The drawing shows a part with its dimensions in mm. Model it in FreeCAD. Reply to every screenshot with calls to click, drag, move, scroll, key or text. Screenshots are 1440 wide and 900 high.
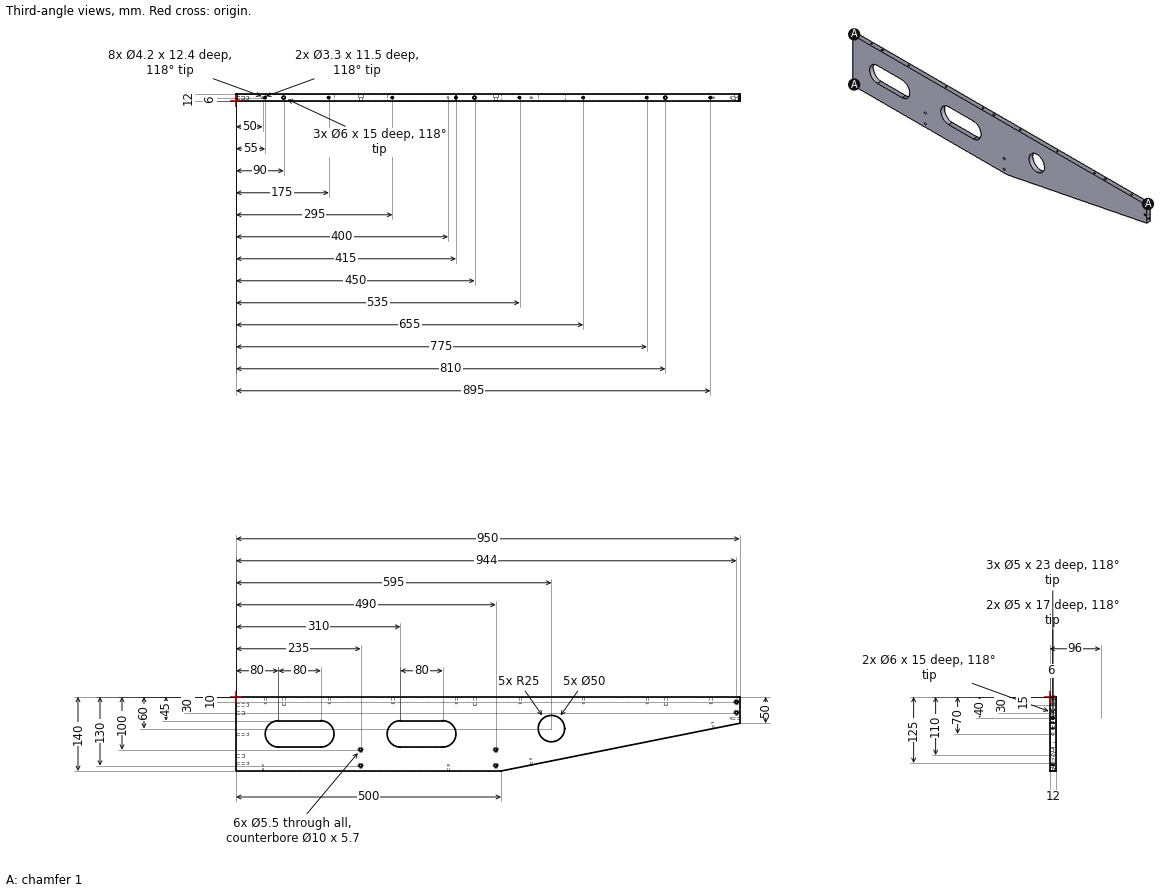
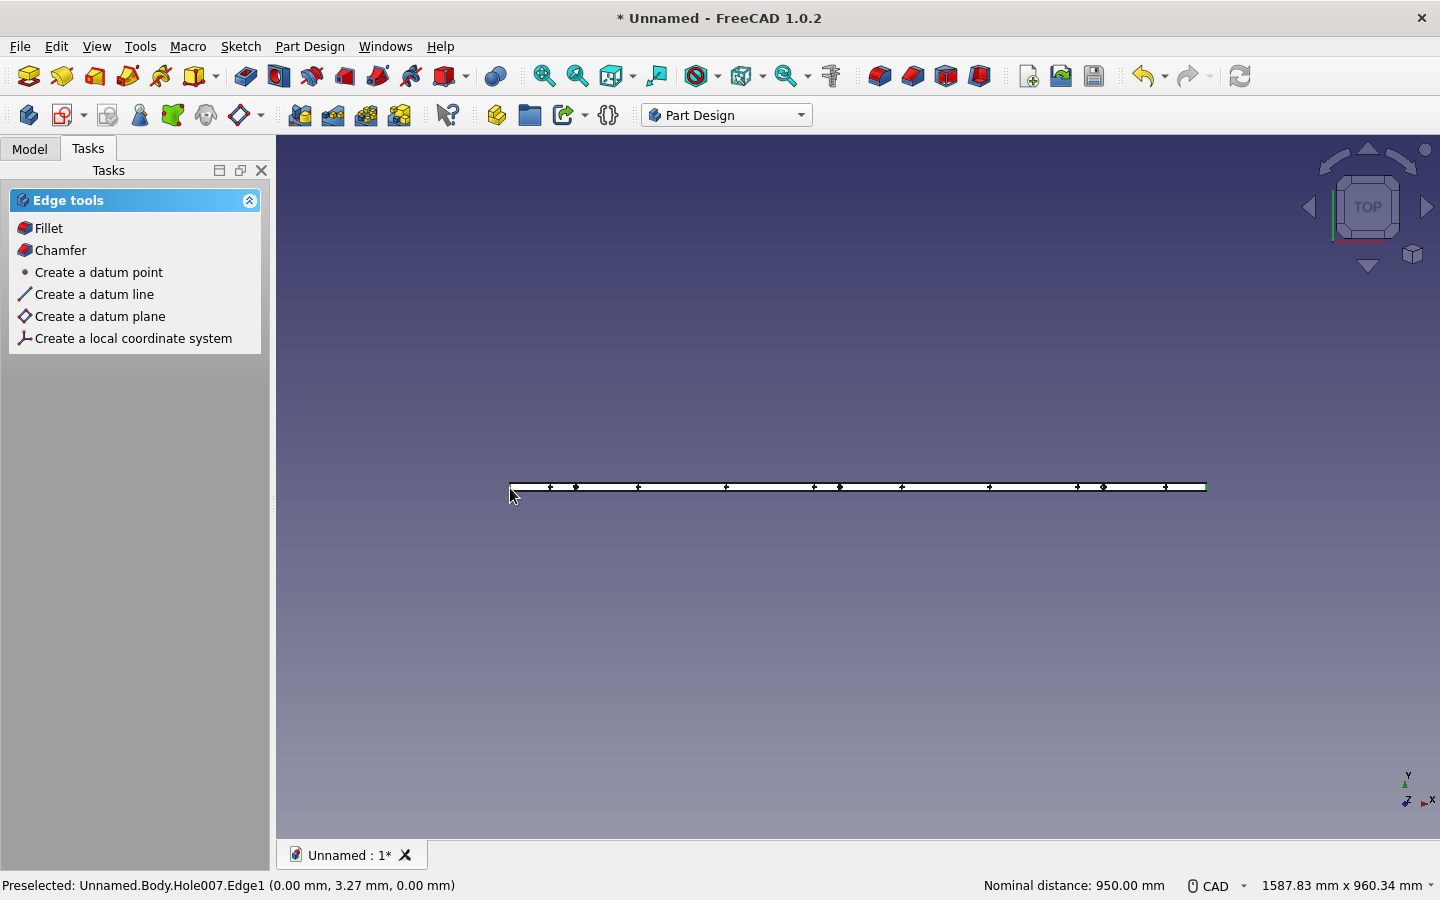
scroll(510, 486, up, 8)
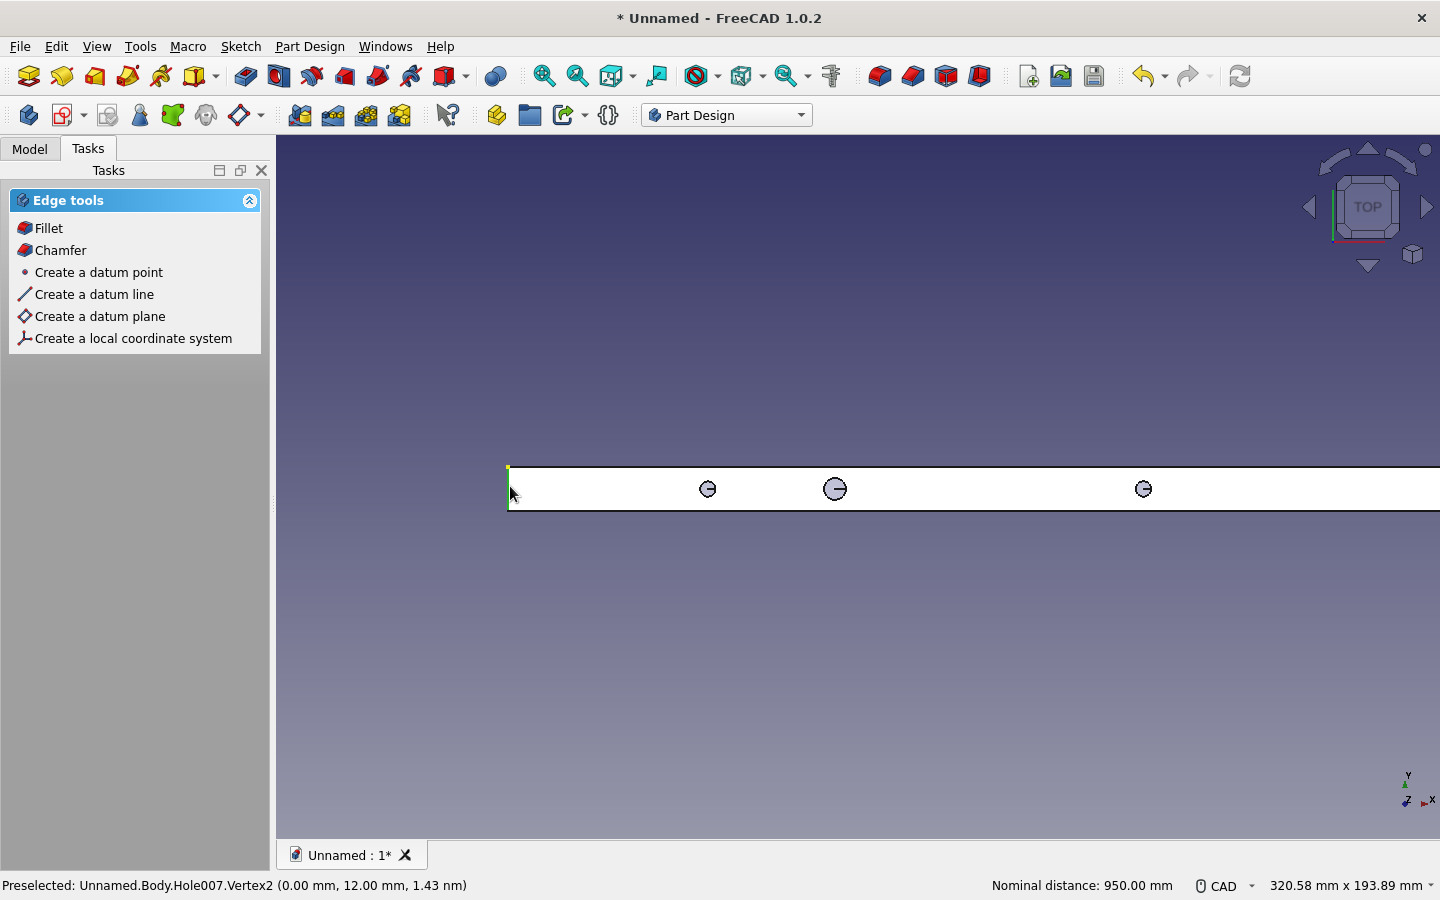
click(545, 76)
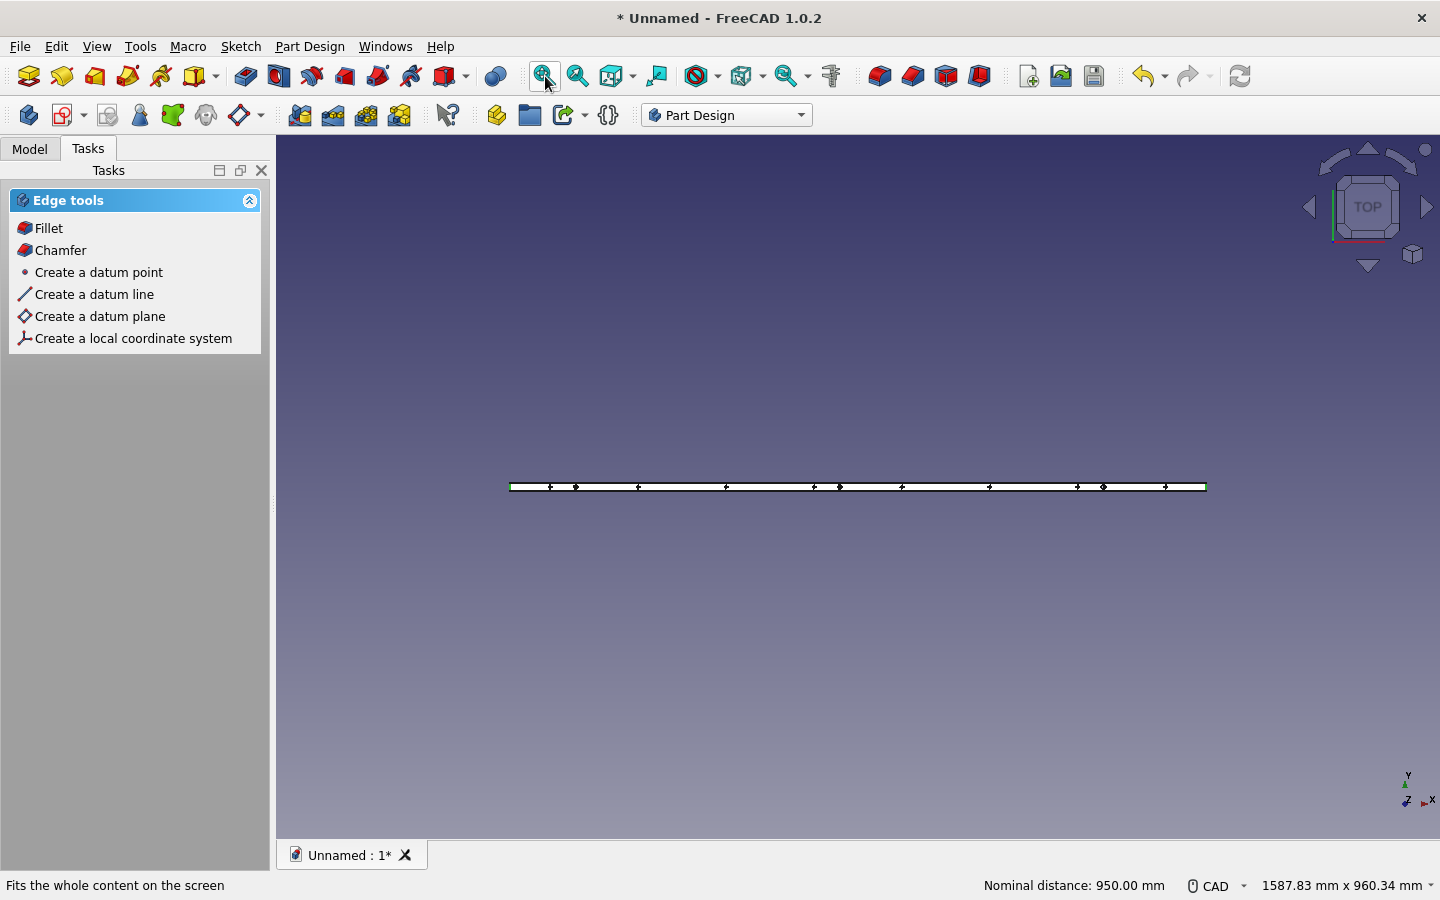
key(1)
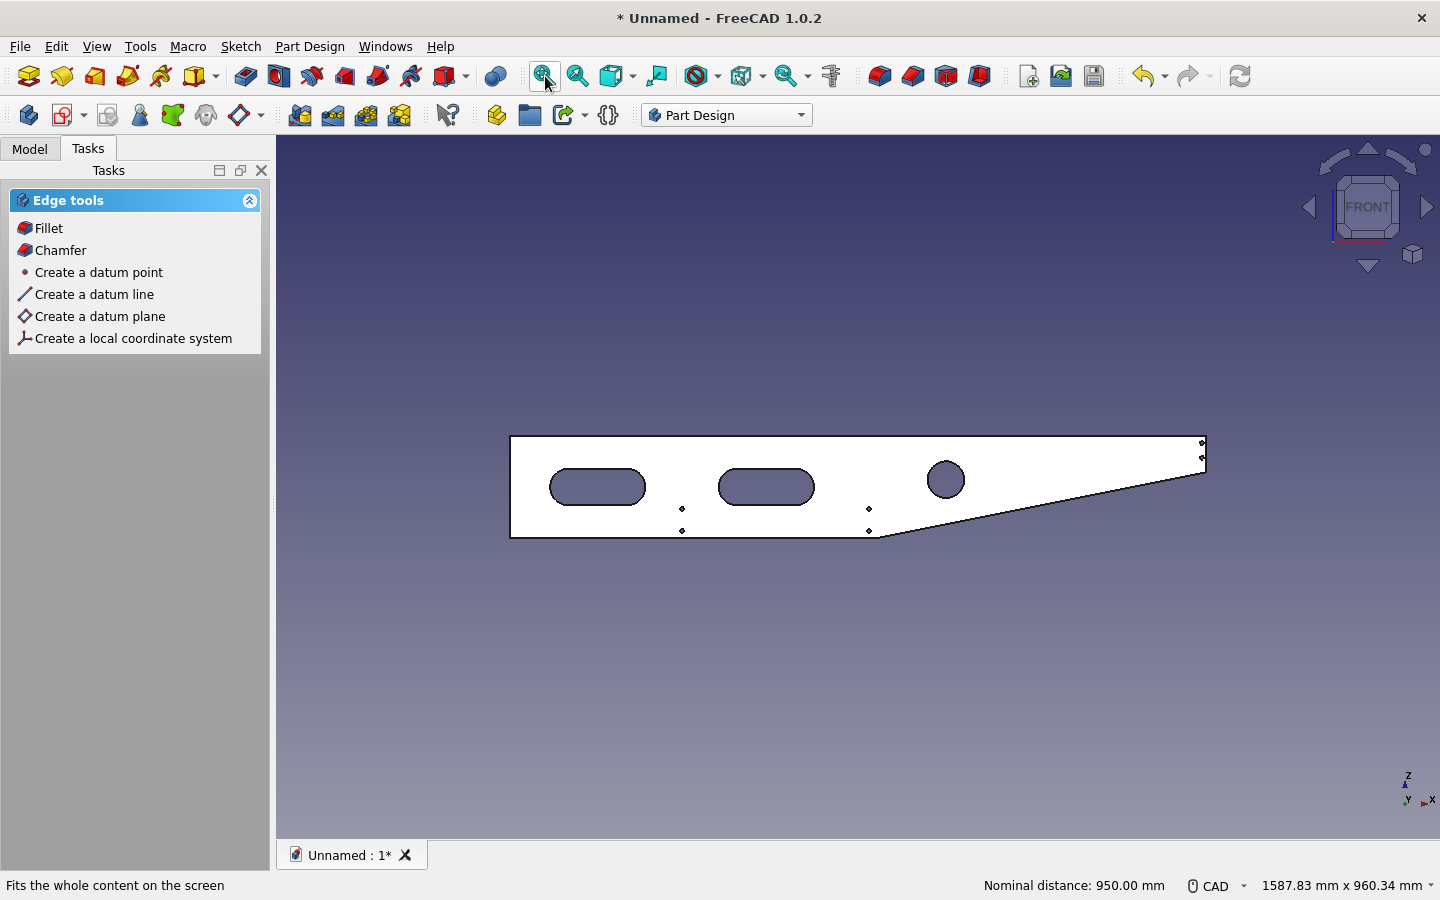
scroll(510, 537, up, 8)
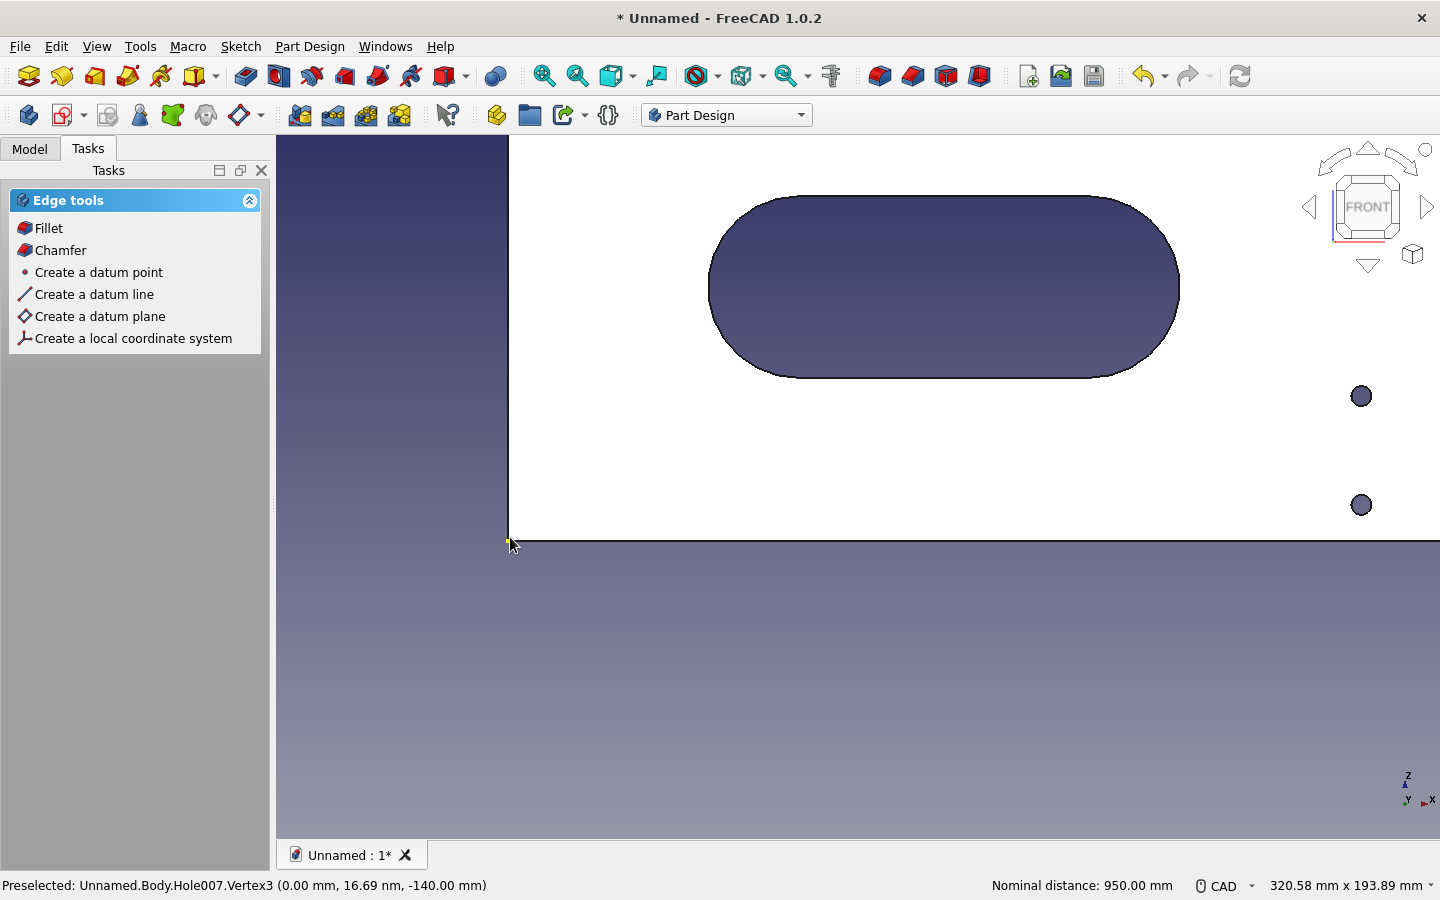
click(545, 76)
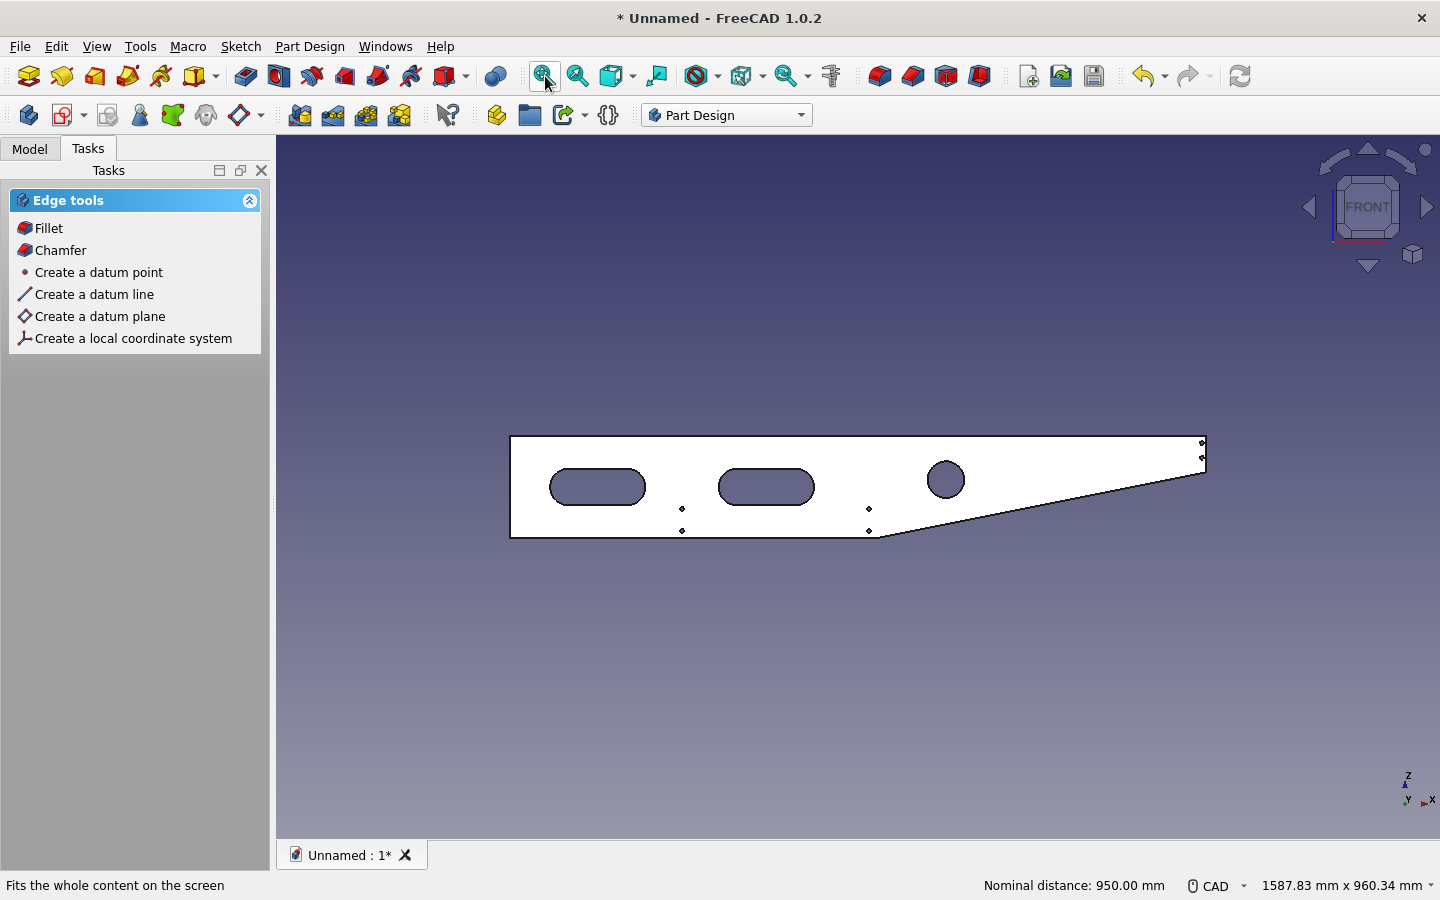
key(3)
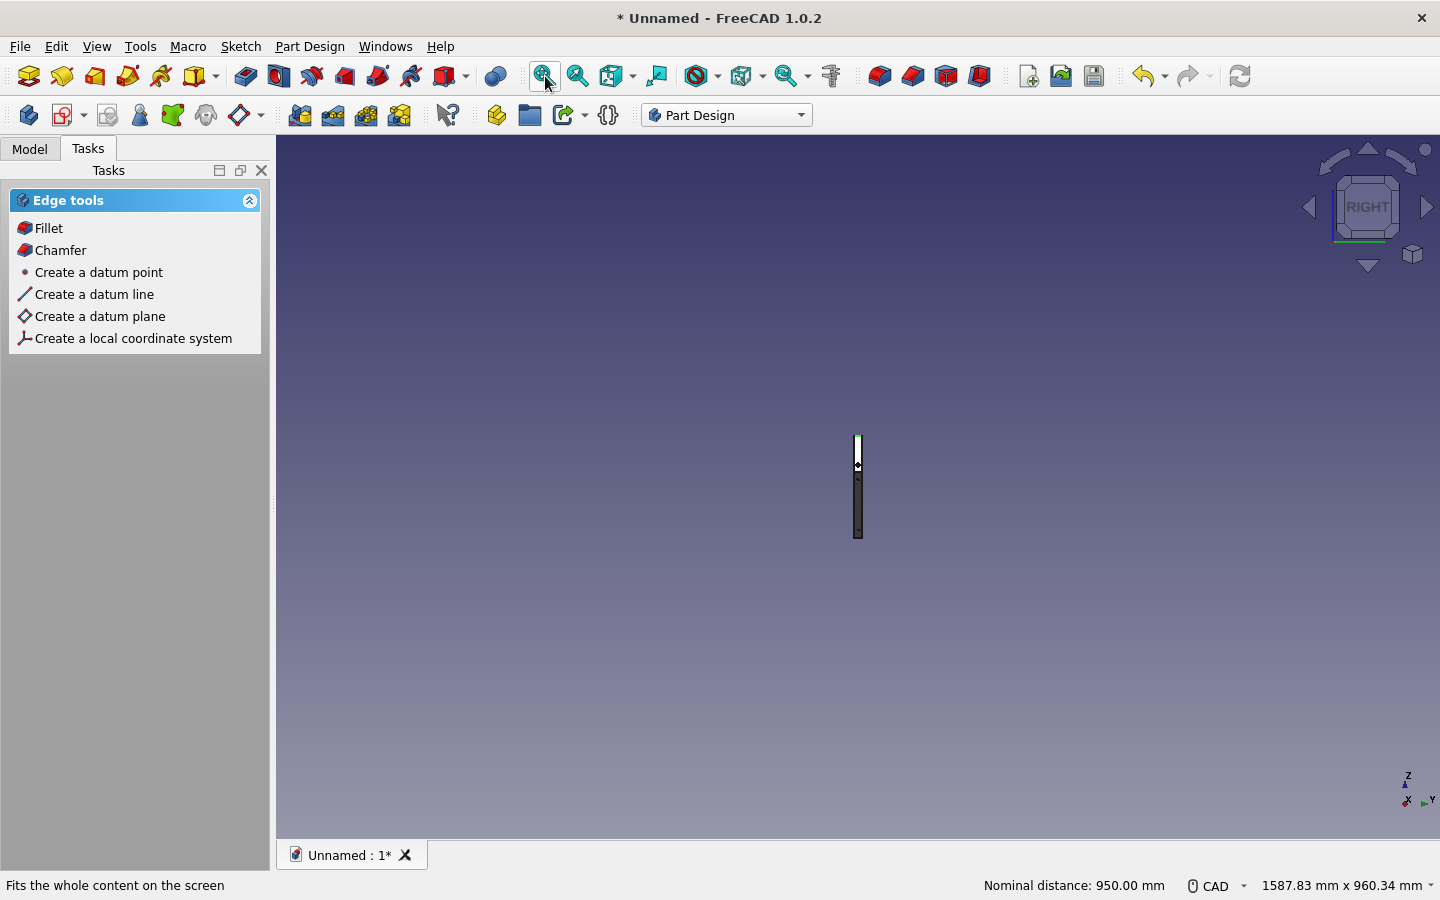
click(545, 76)